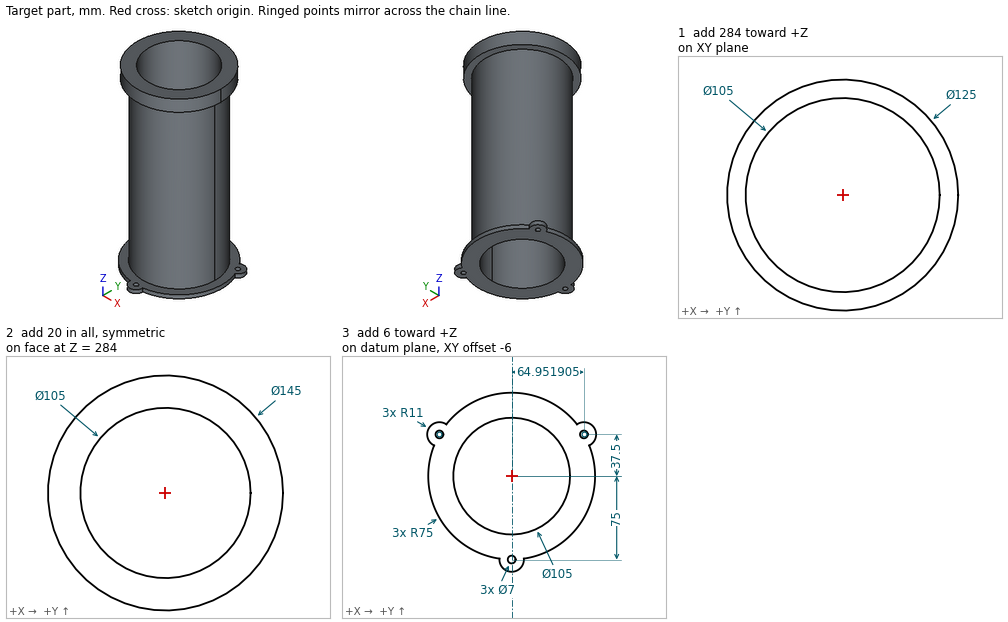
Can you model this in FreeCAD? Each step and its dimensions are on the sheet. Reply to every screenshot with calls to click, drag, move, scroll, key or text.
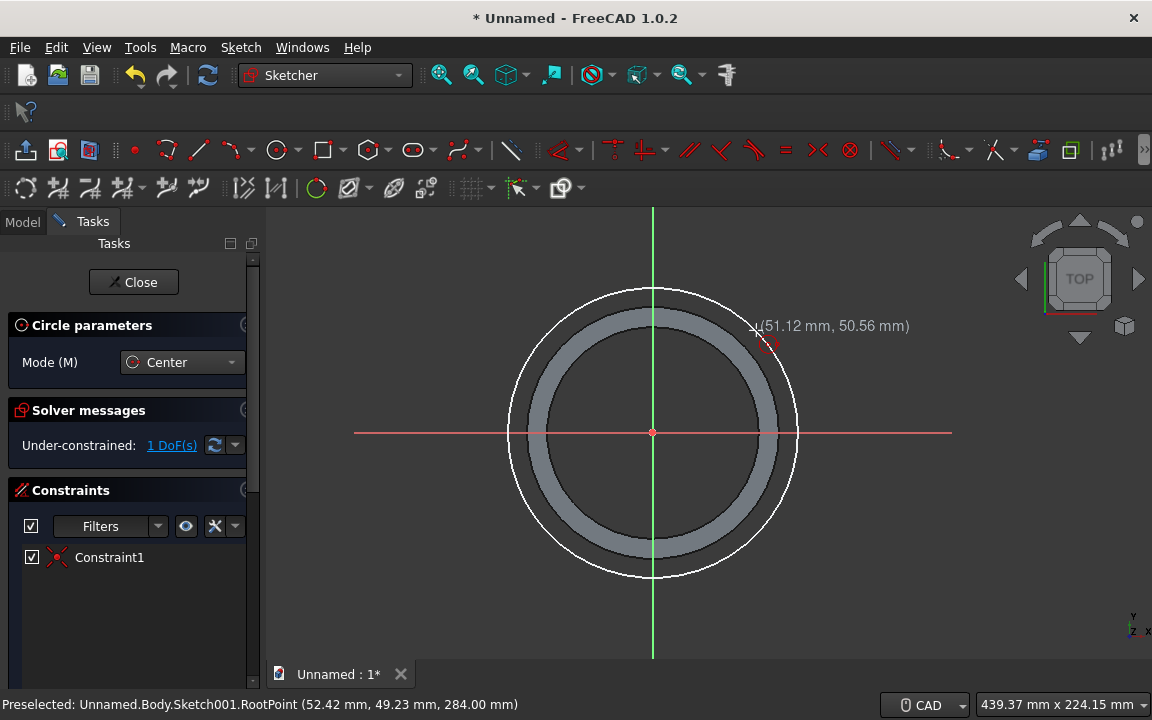
click(653, 433)
click(728, 358)
key(Escape)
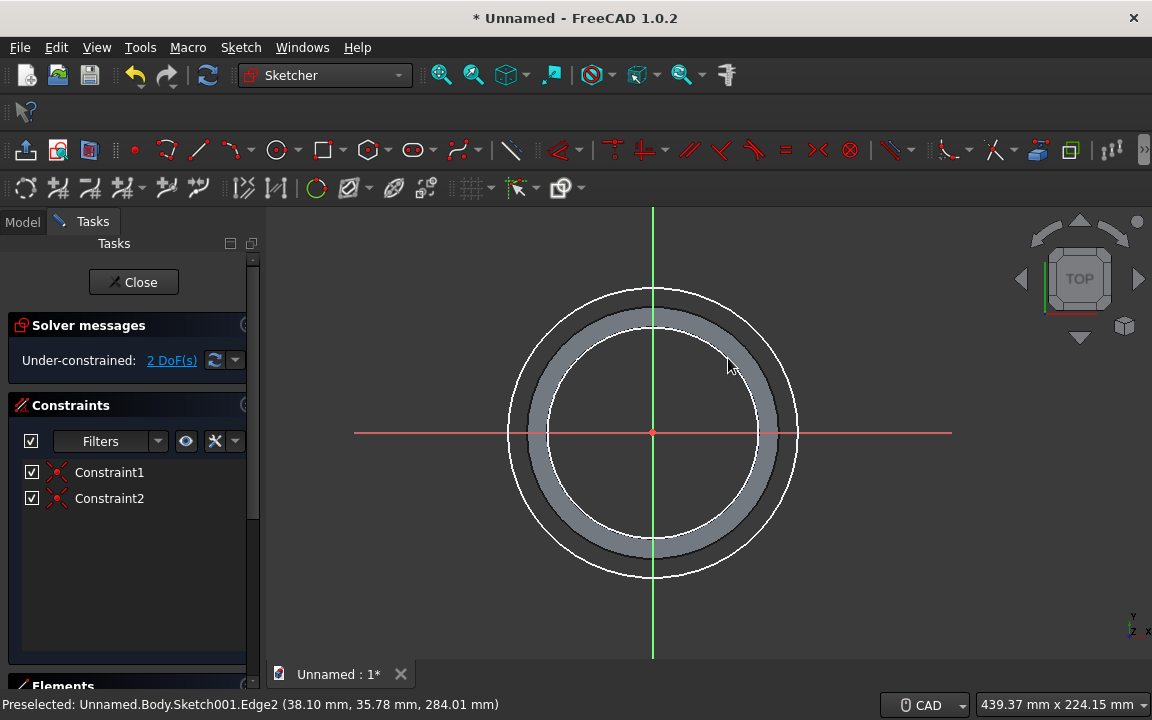
key(d)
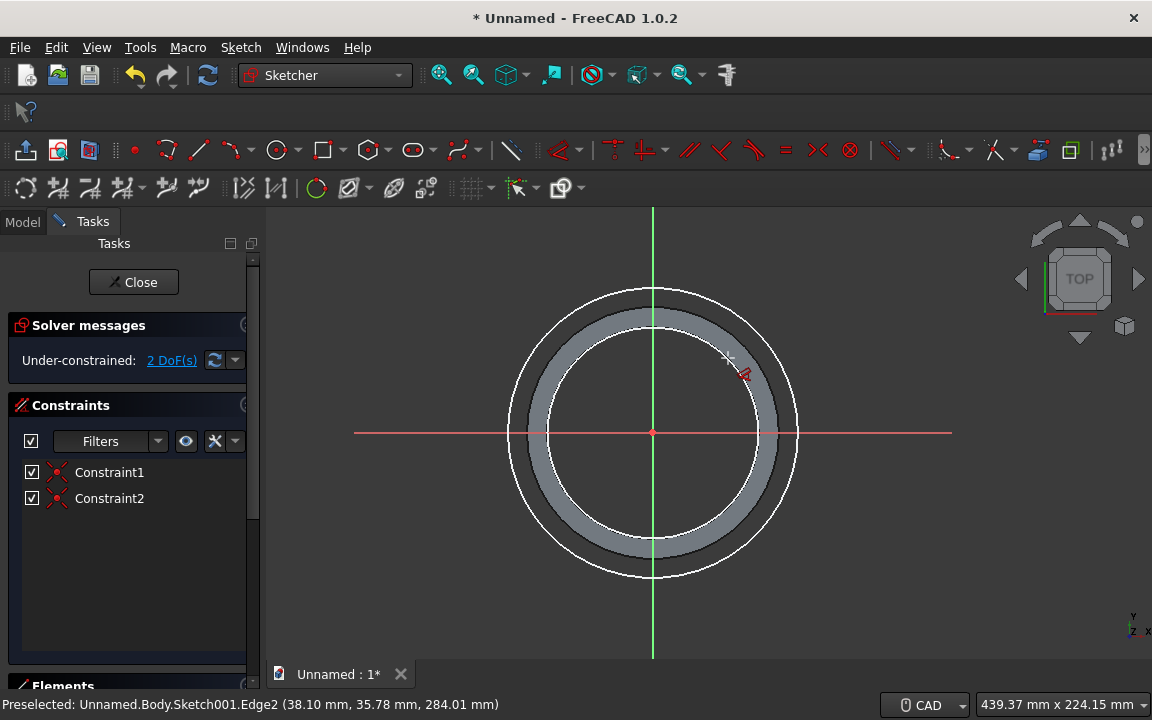
click(755, 330)
click(778, 307)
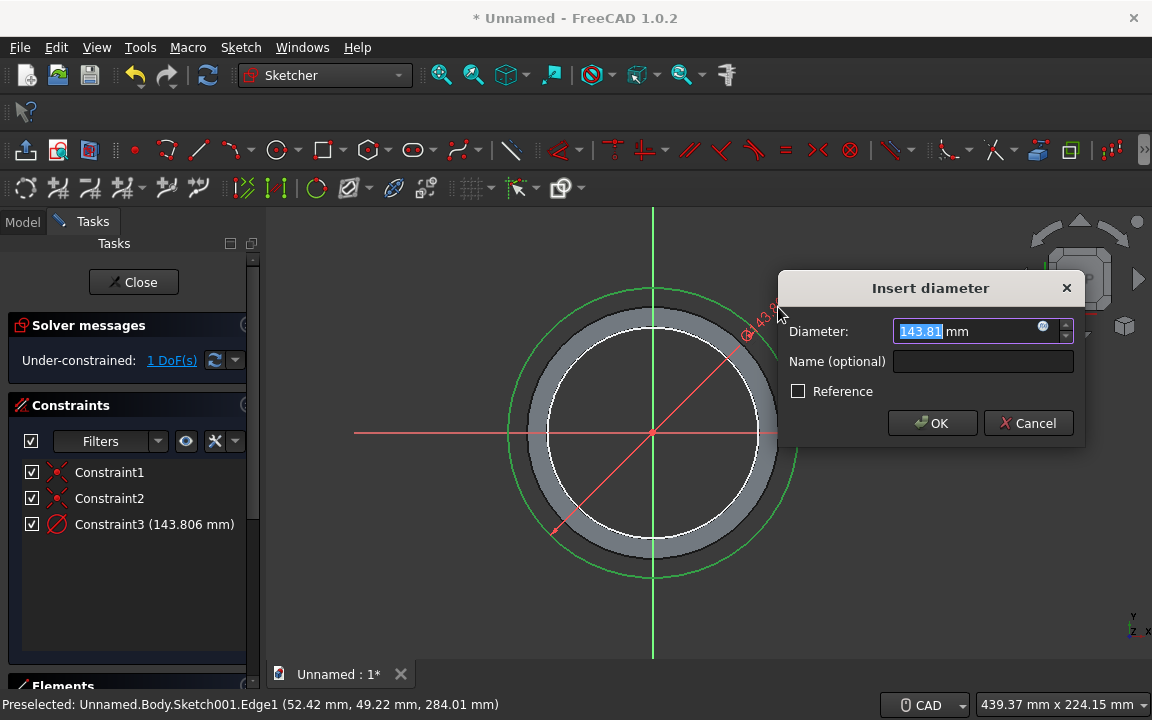
text(145)
key(Return)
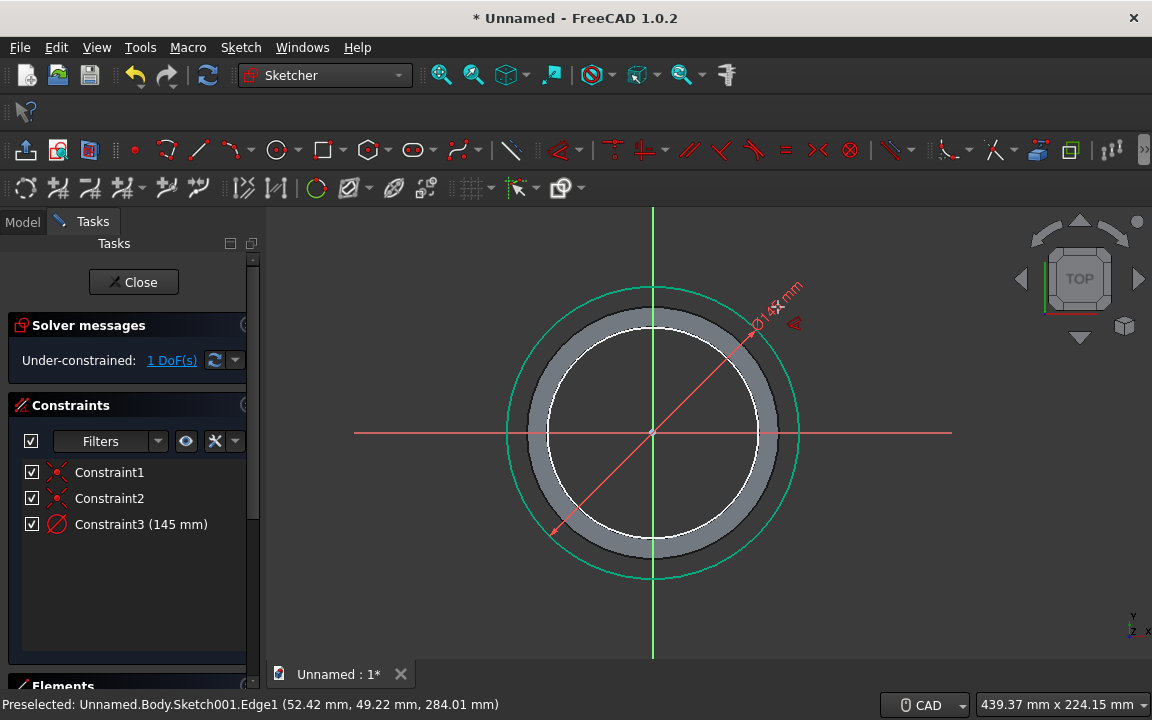
click(727, 358)
click(807, 387)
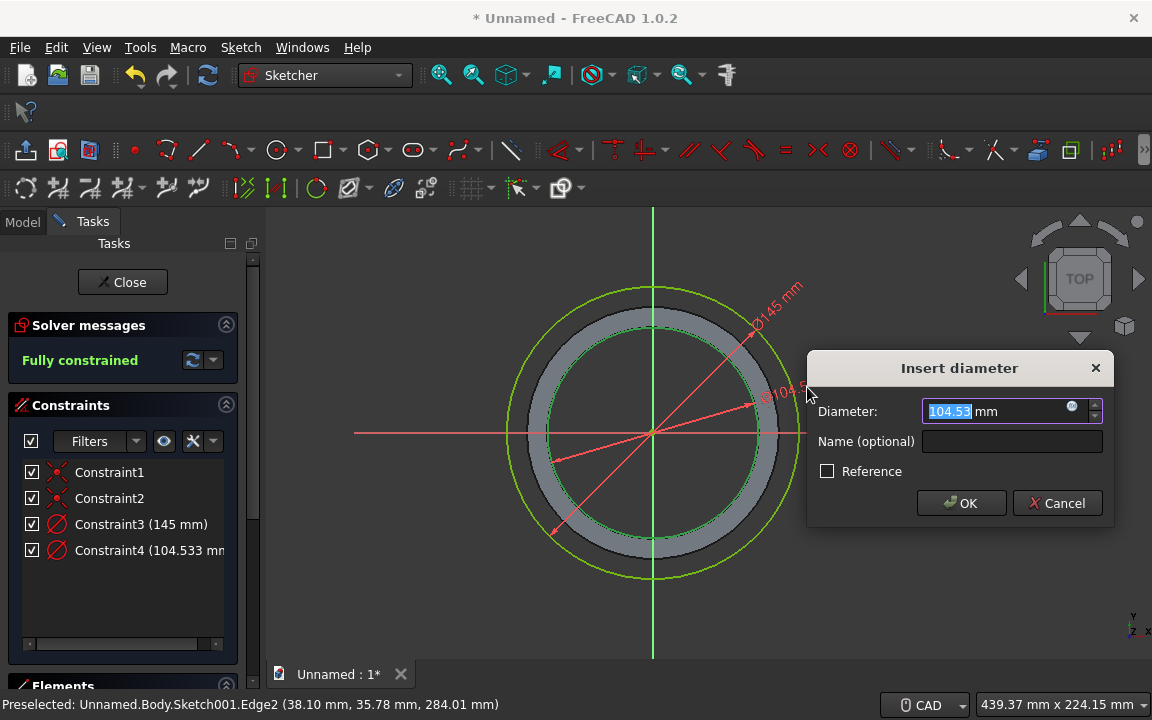
text(105)
key(Return)
key(Escape)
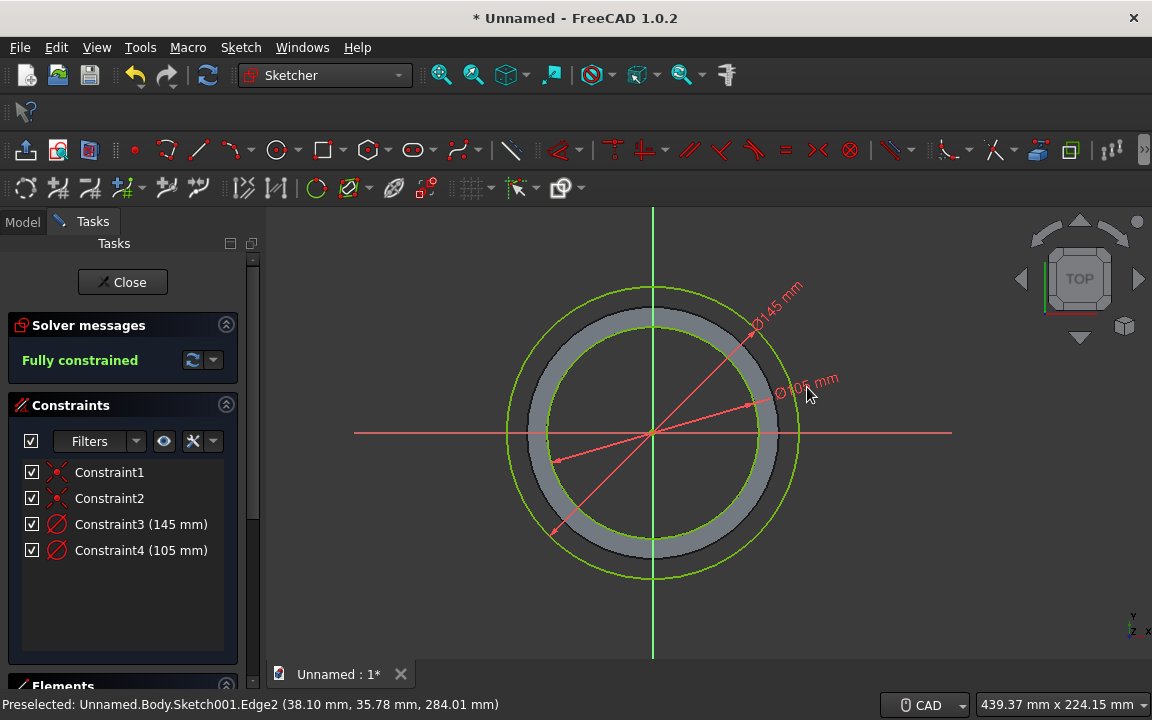
click(123, 282)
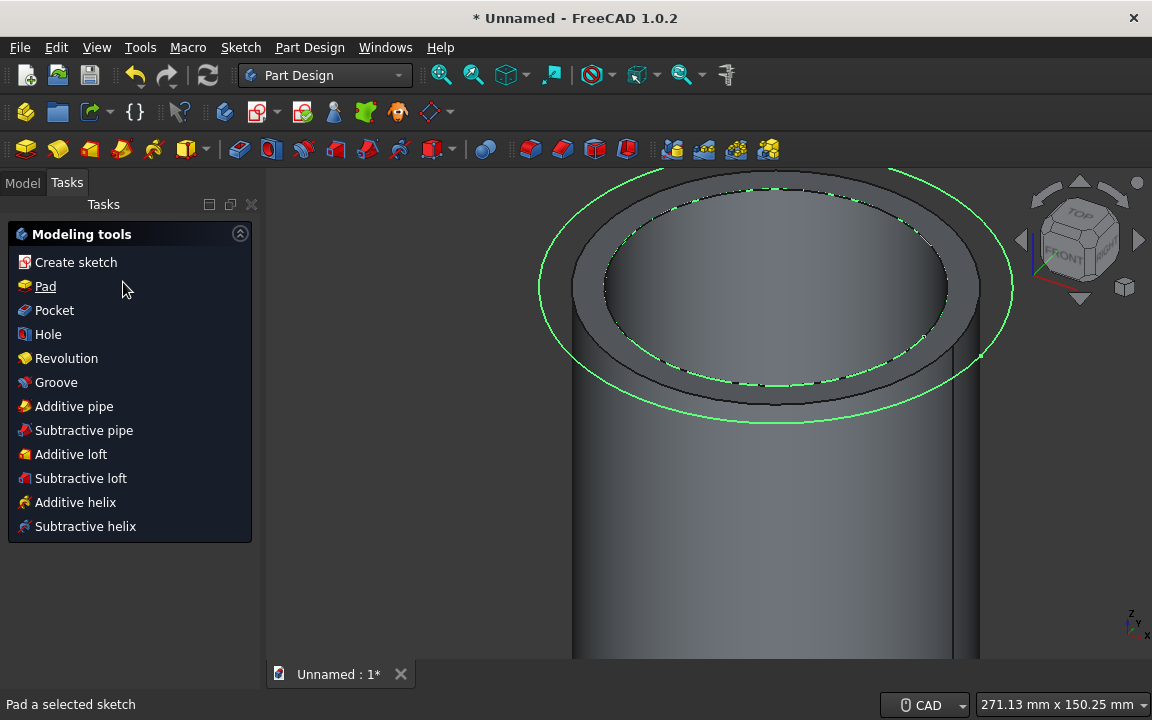
click(26, 150)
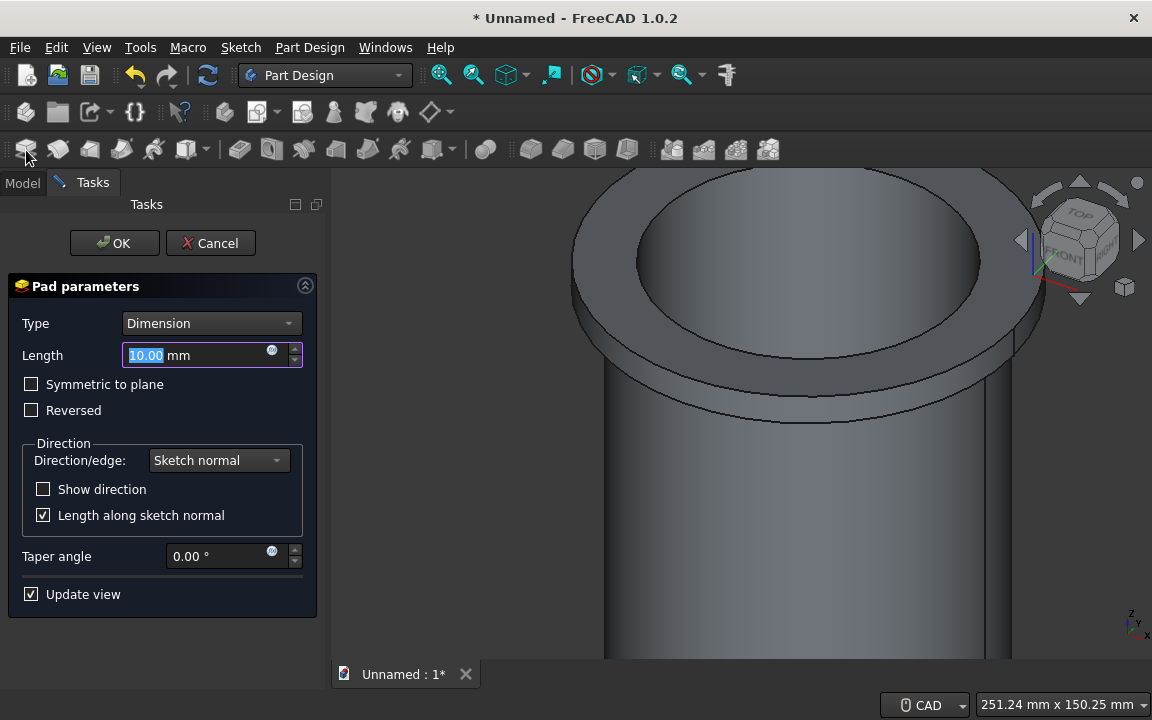
text(20)
key(Tab)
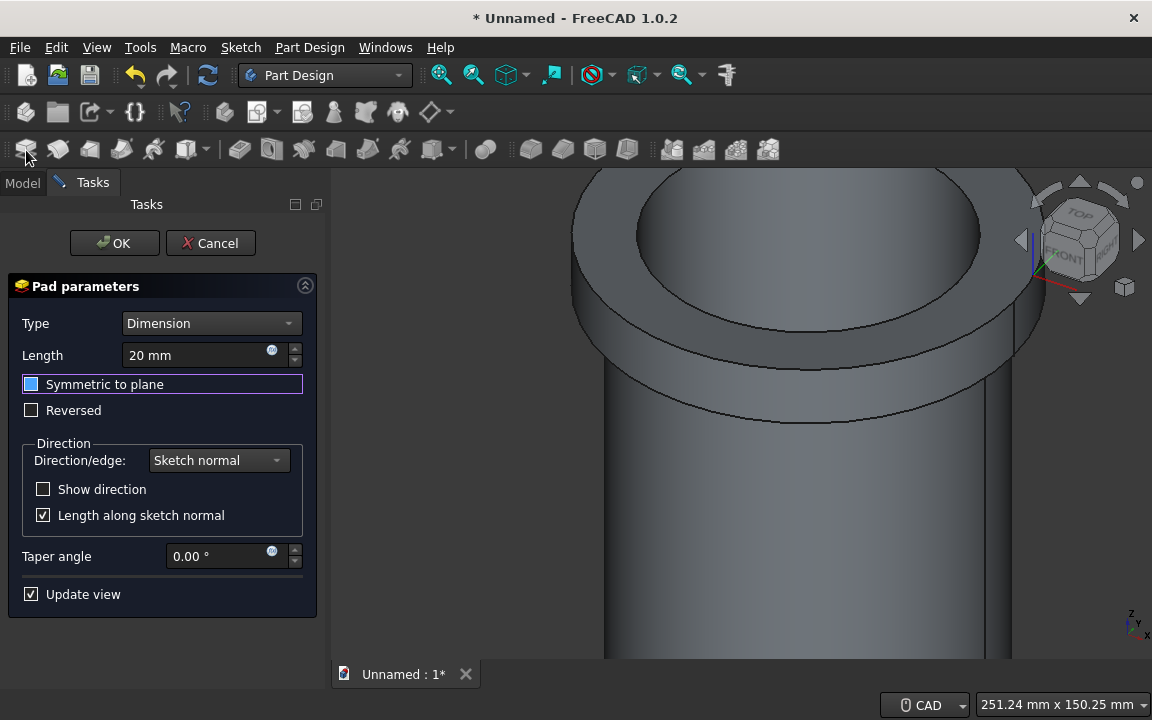
click(30, 384)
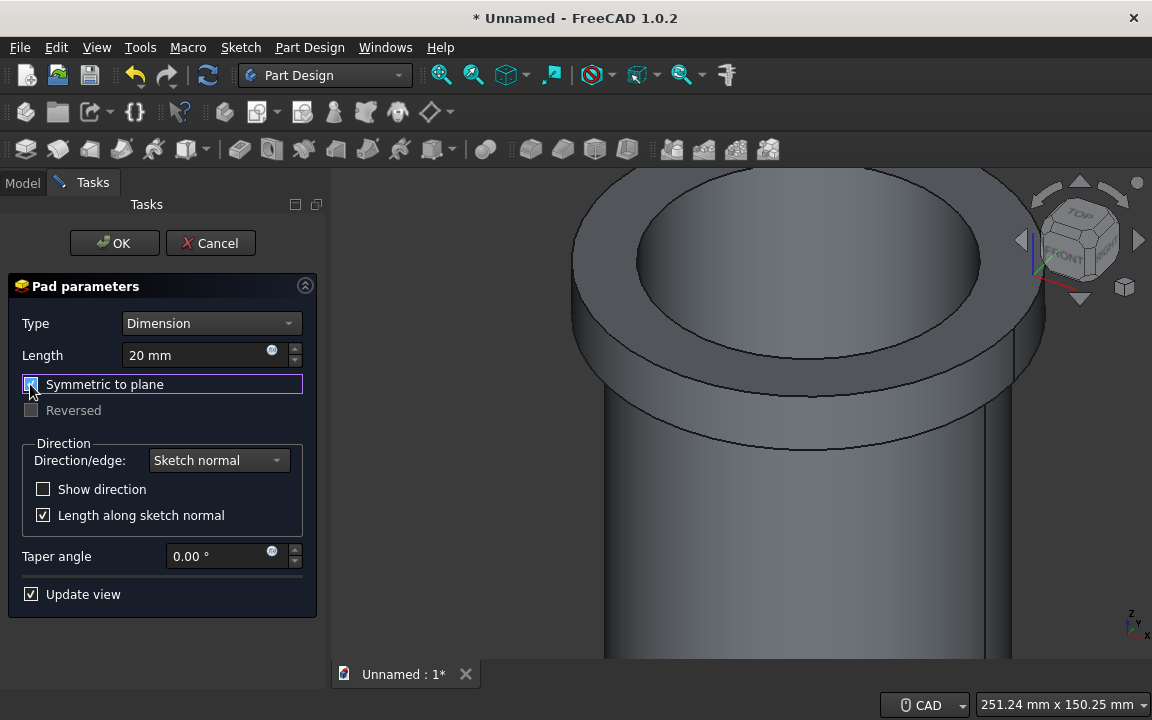
click(115, 243)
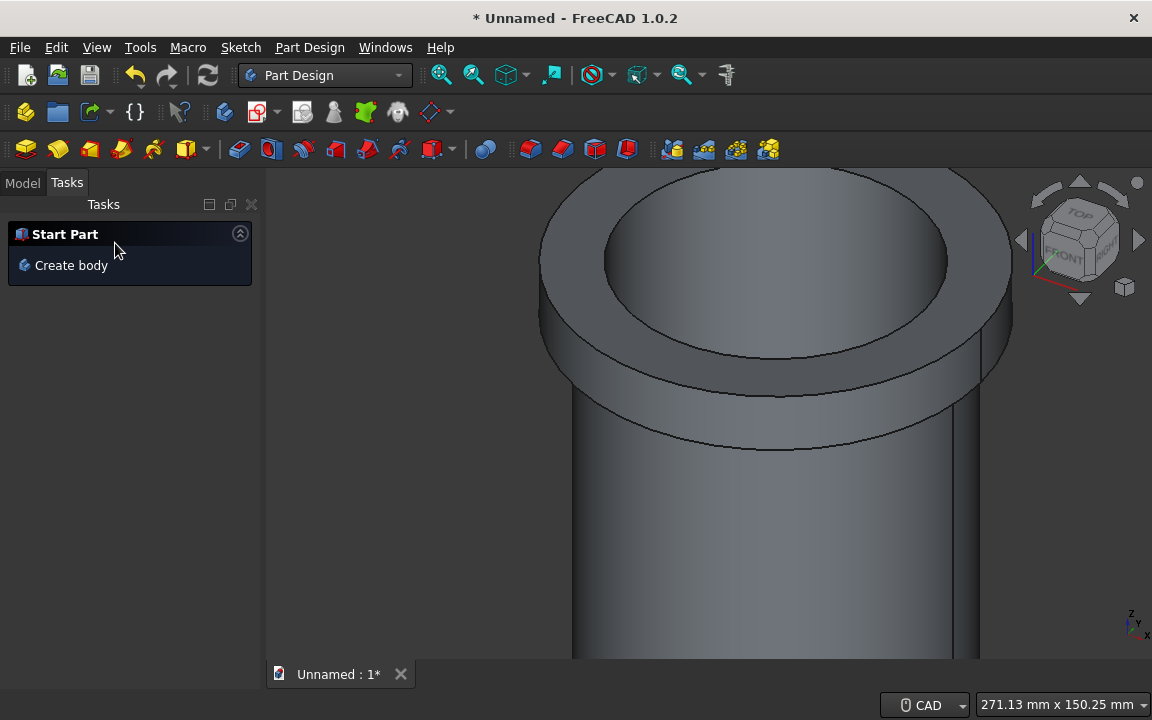
click(442, 76)